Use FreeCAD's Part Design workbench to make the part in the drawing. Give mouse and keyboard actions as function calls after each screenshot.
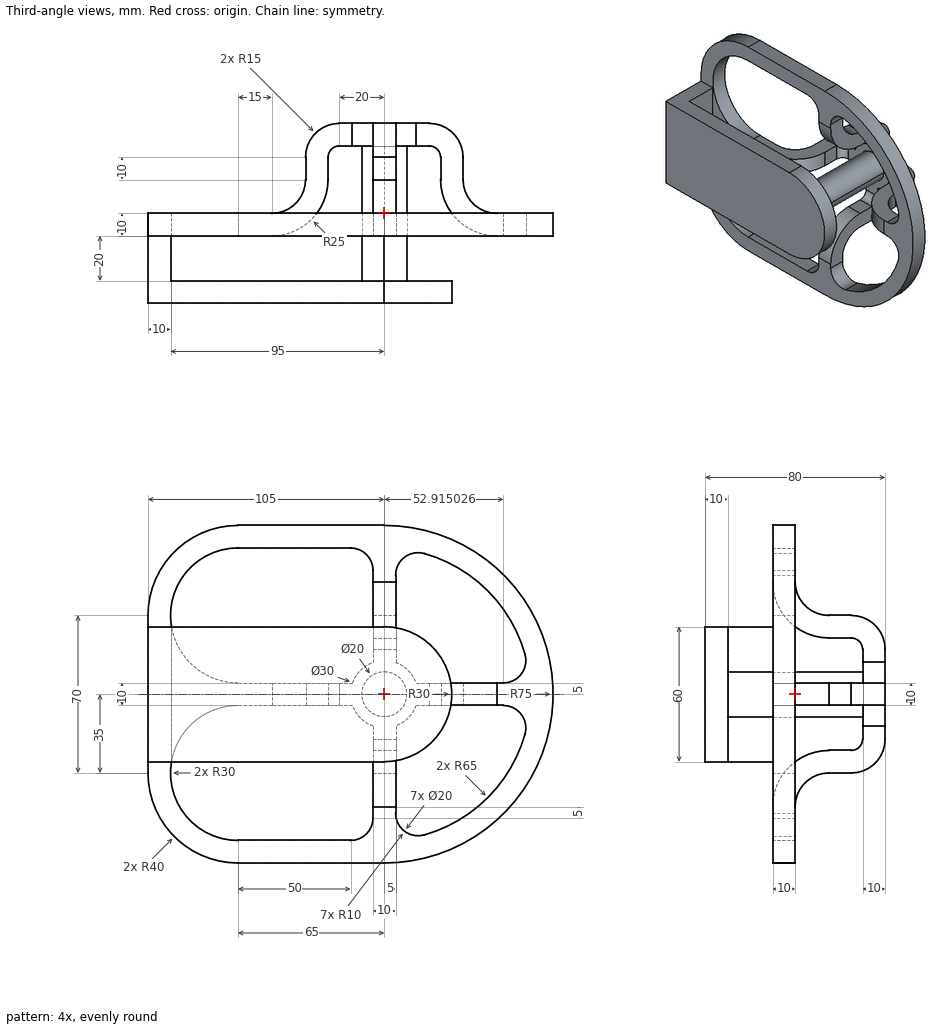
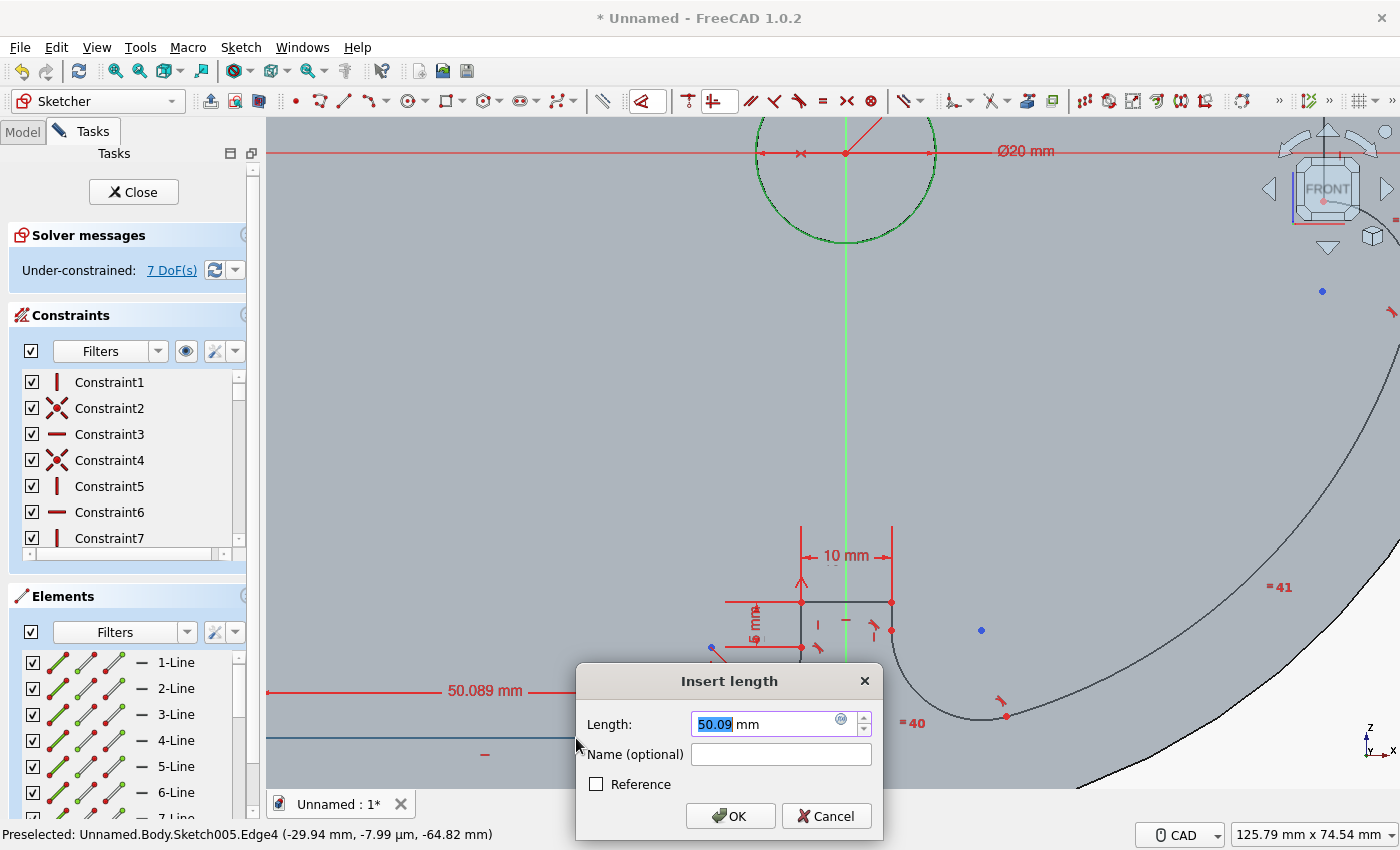
text(50)
key(Return)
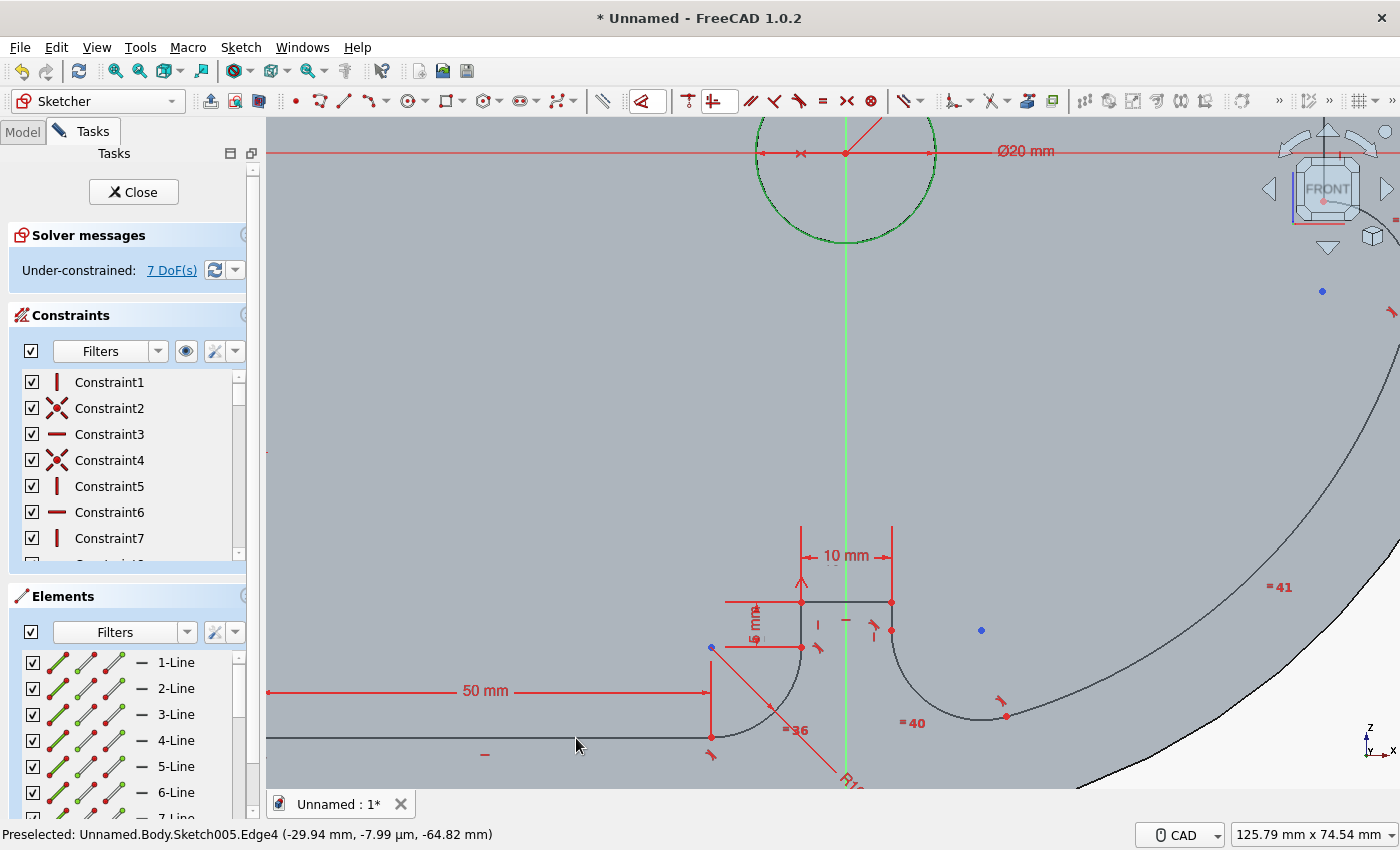
scroll(802, 627, down, 5)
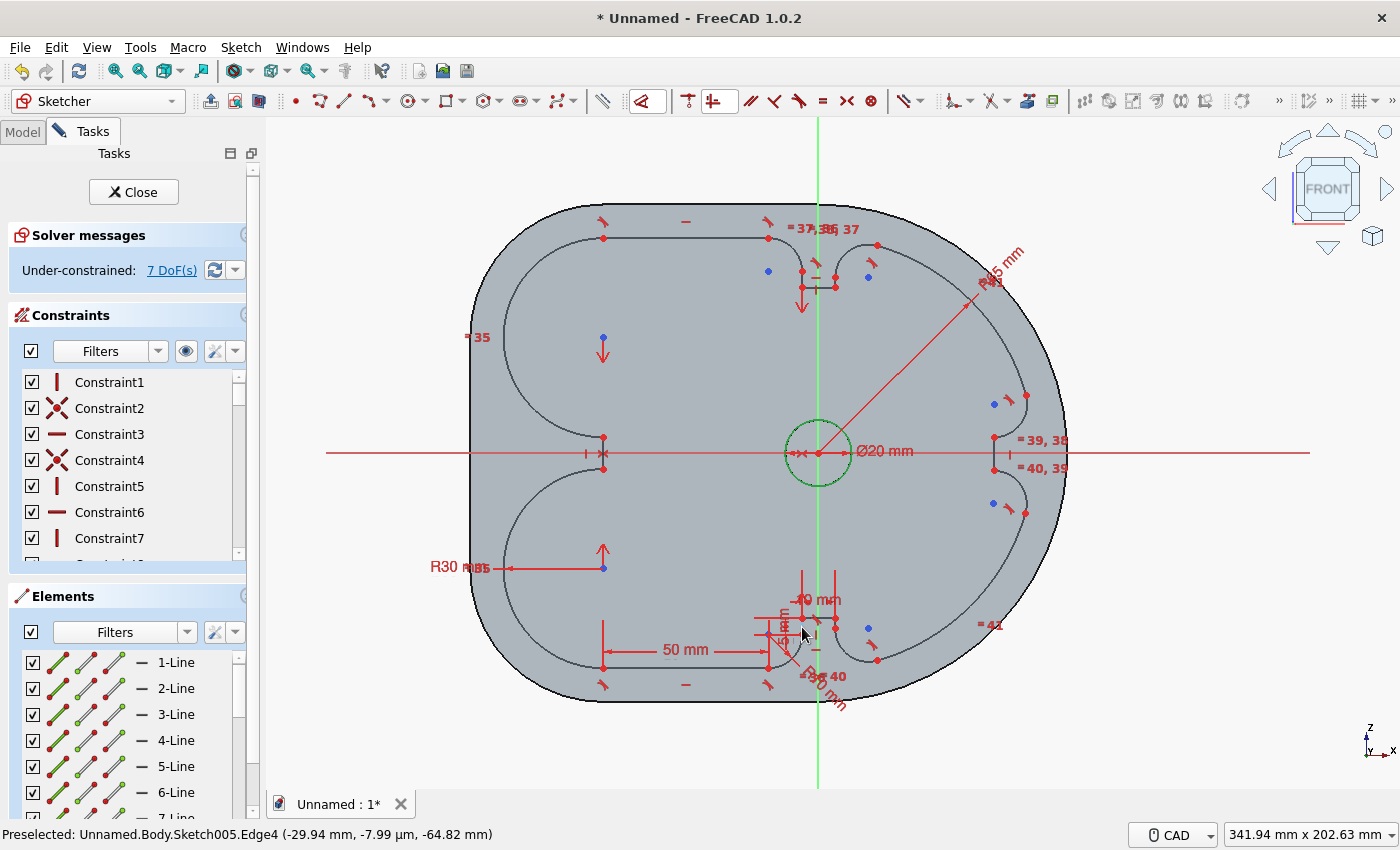
scroll(603, 460, up, 4)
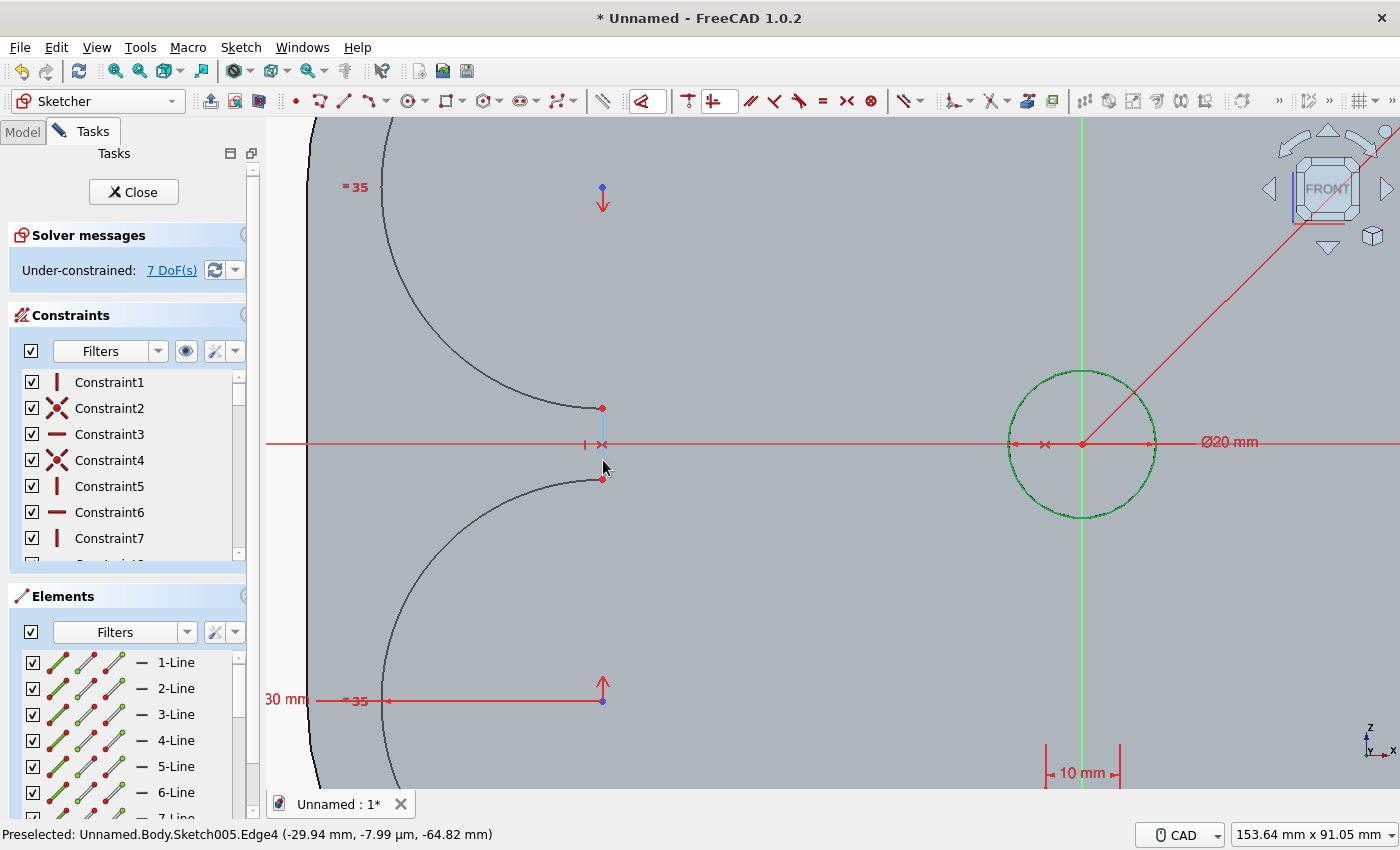
click(603, 458)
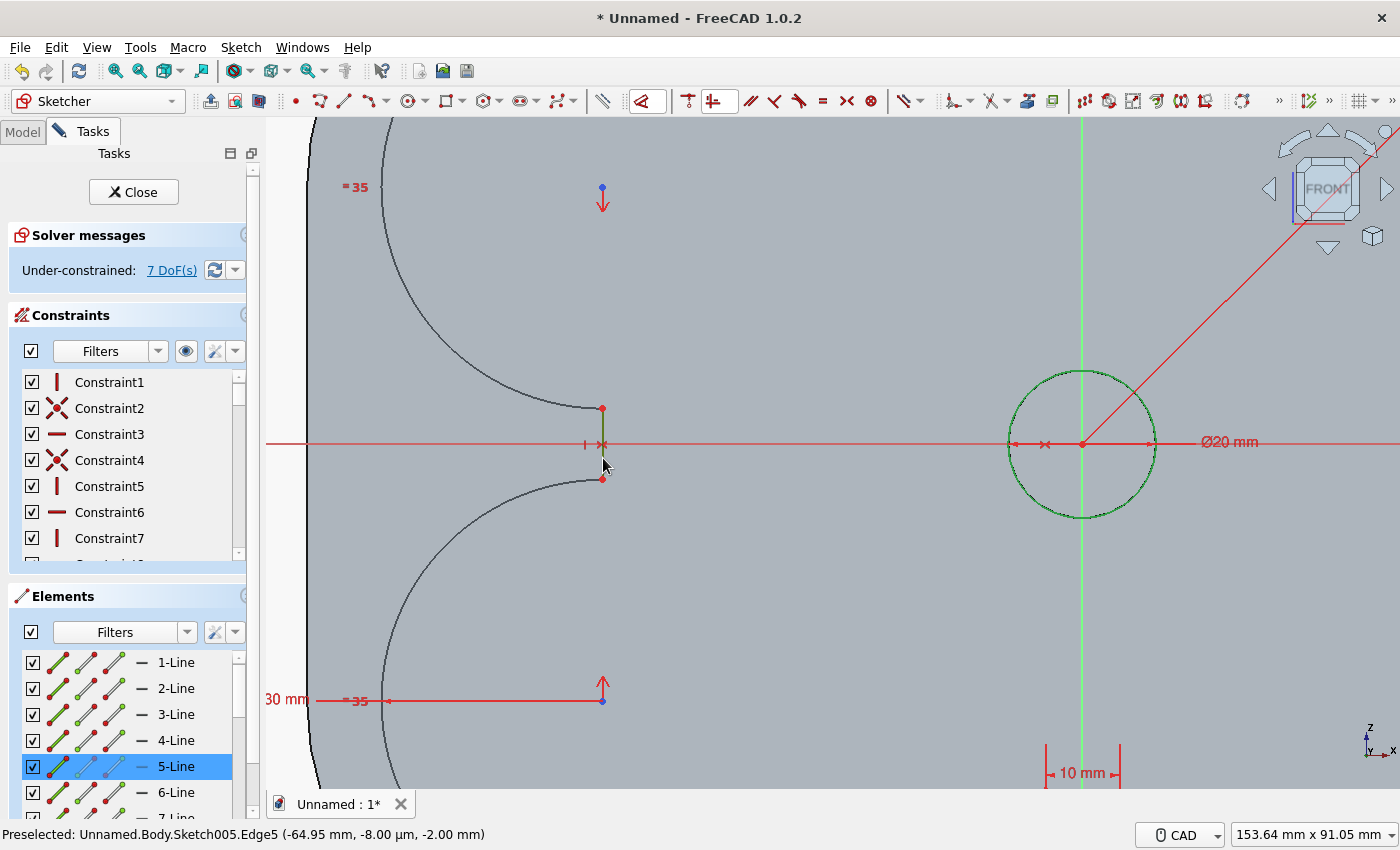
click(660, 102)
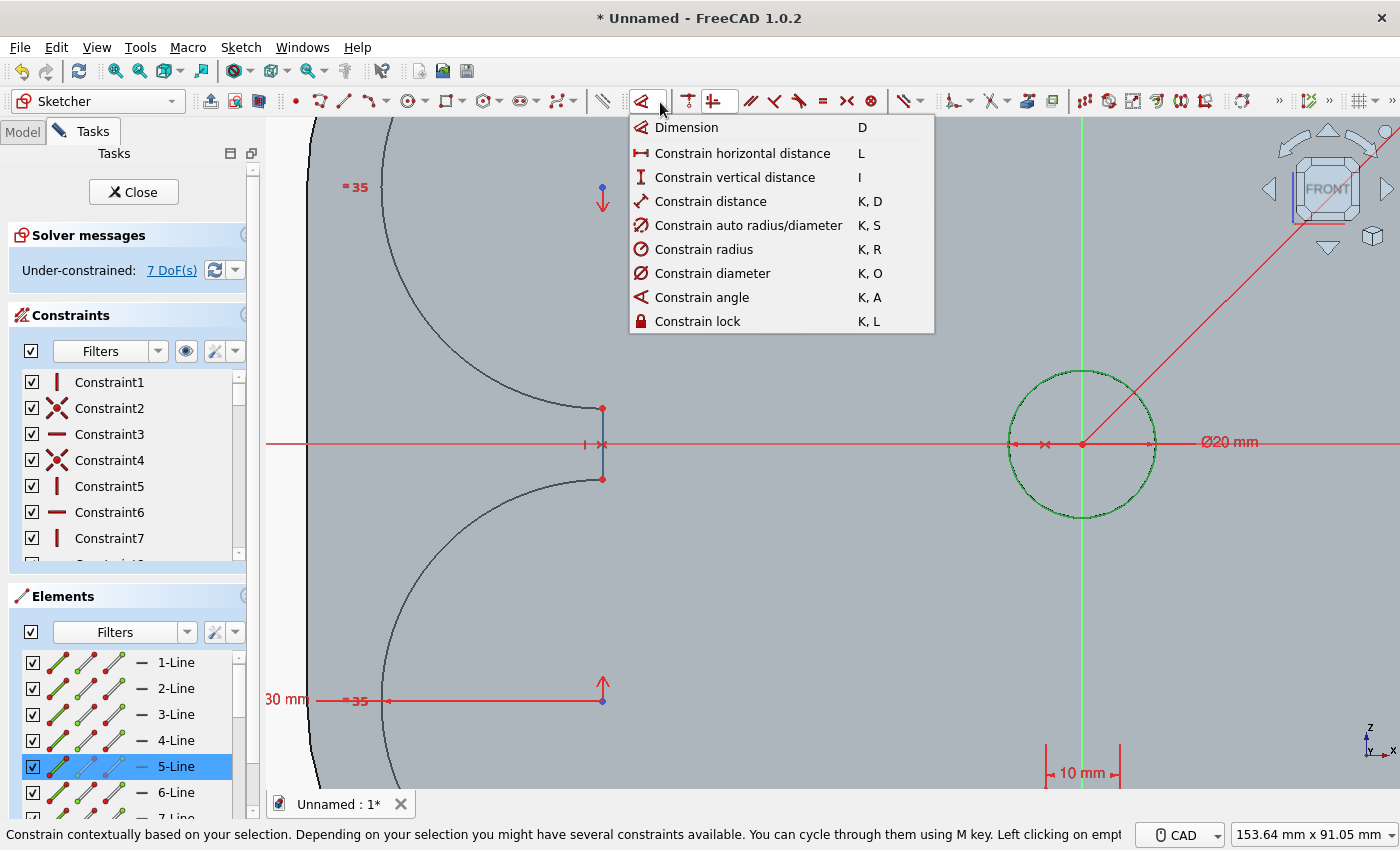
click(782, 177)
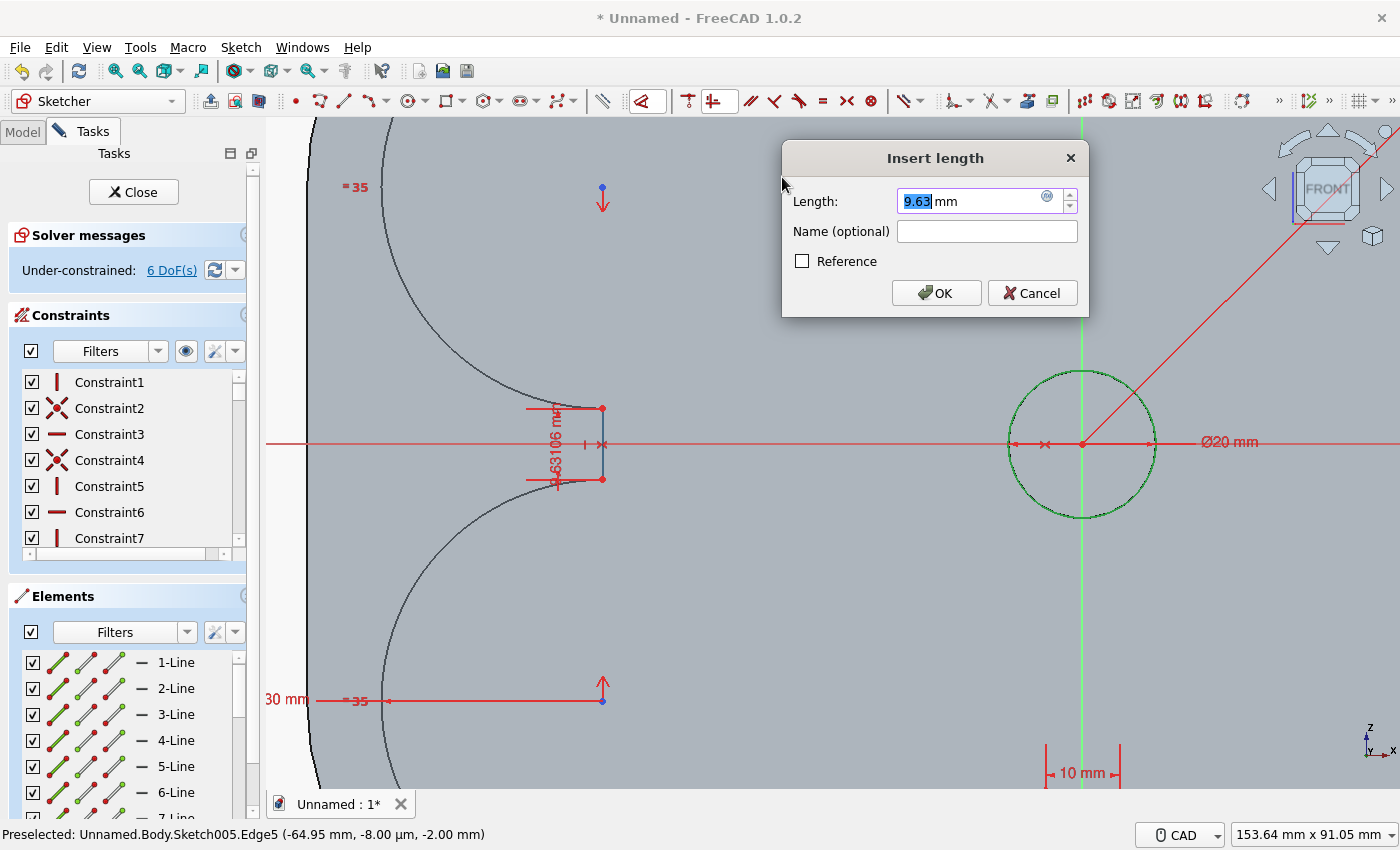
text(10)
key(Return)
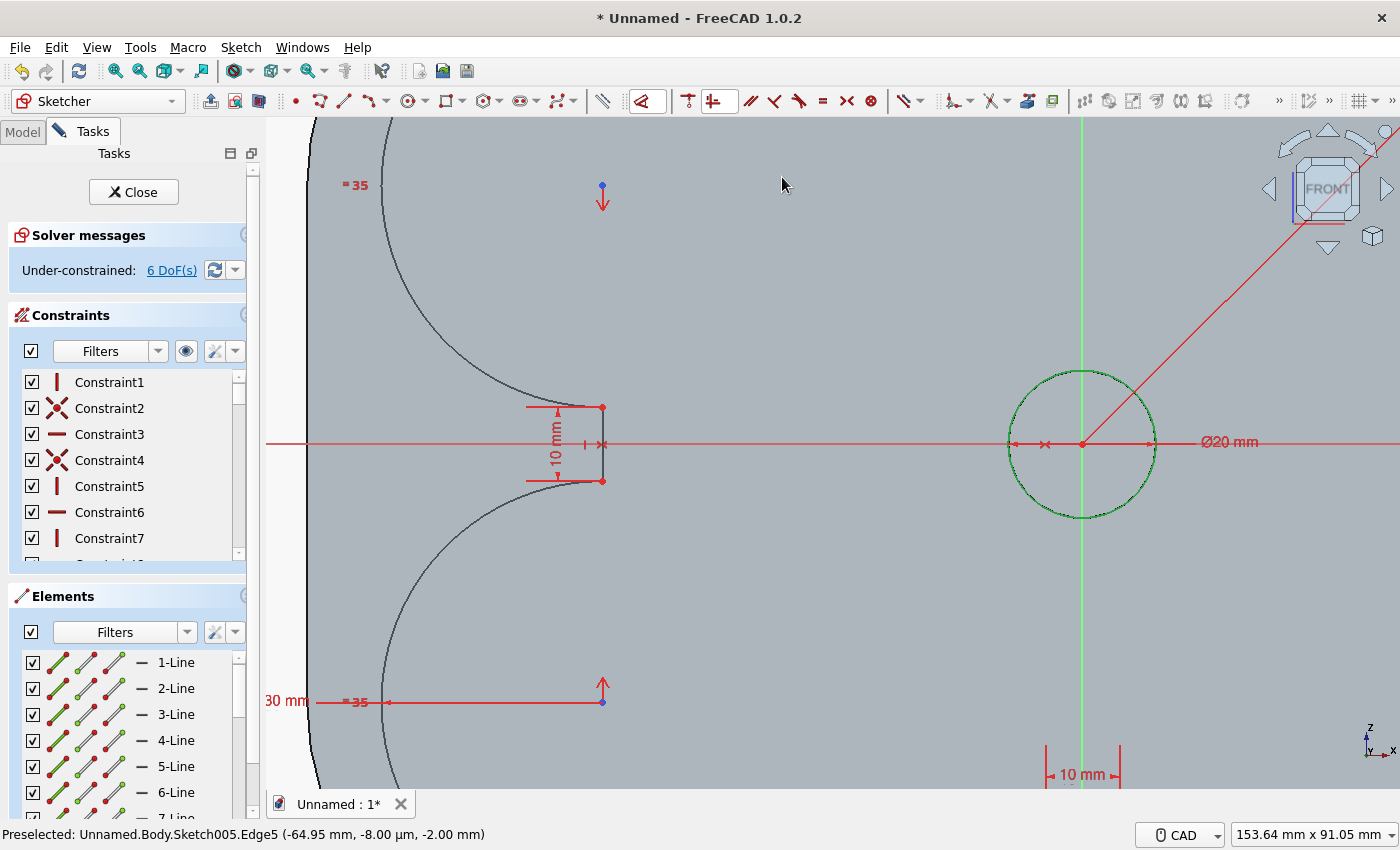
scroll(603, 460, down, 4)